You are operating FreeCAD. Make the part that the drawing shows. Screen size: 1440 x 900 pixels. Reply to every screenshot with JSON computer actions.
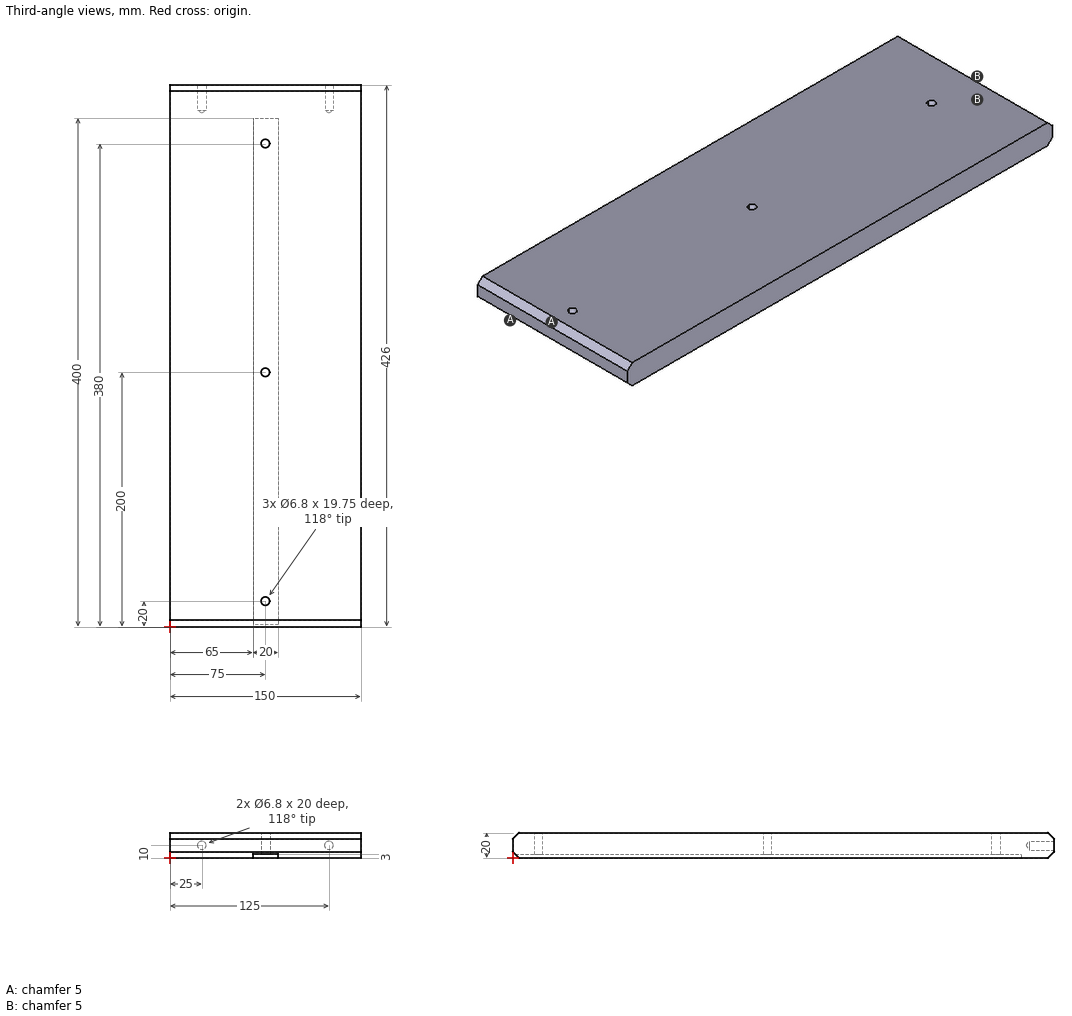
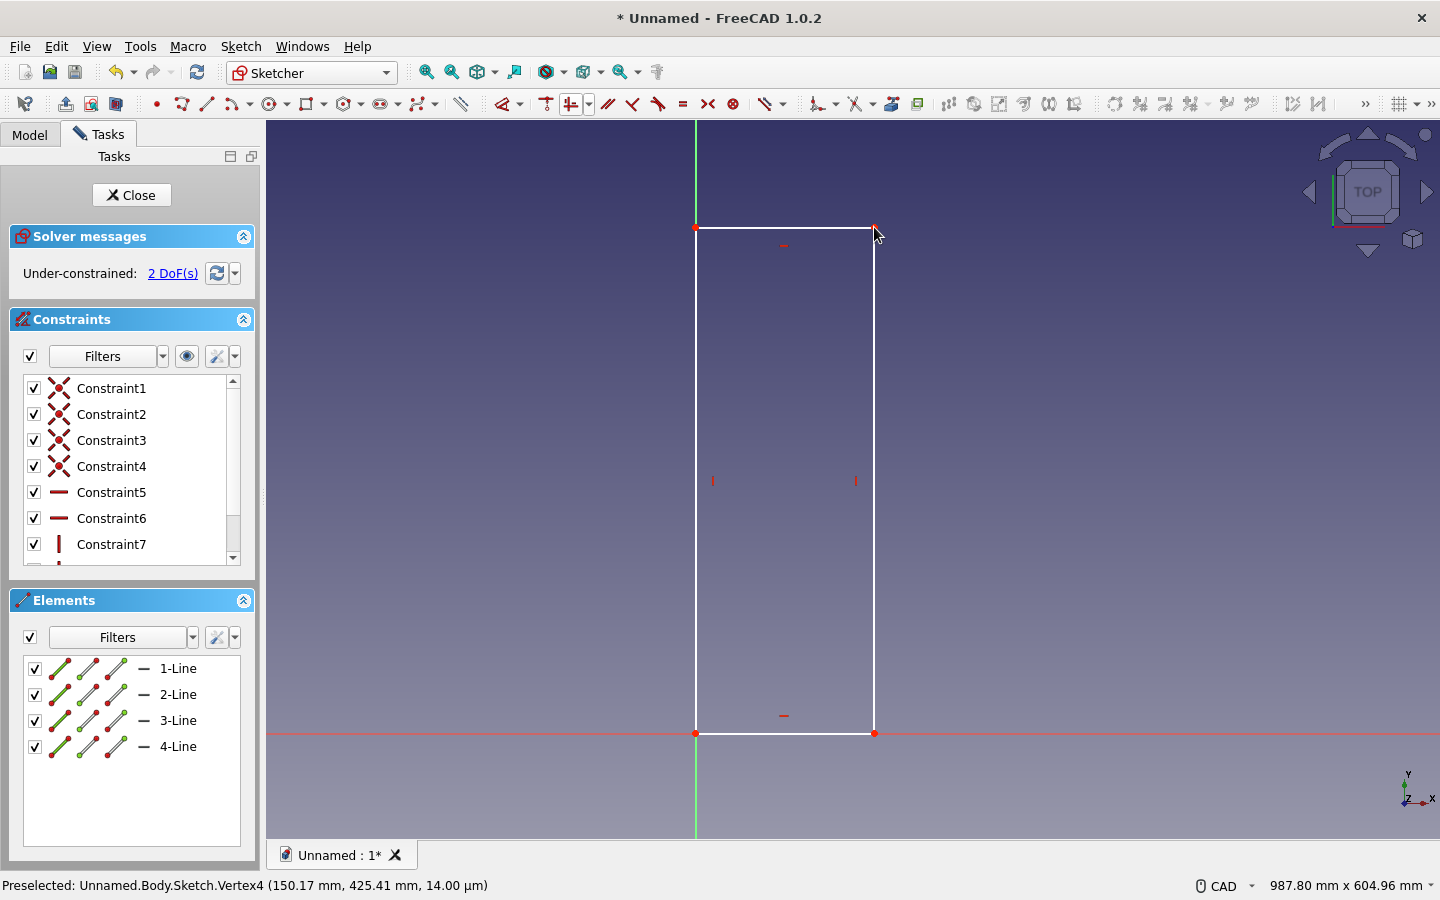
{"action": "key", "text": "d"}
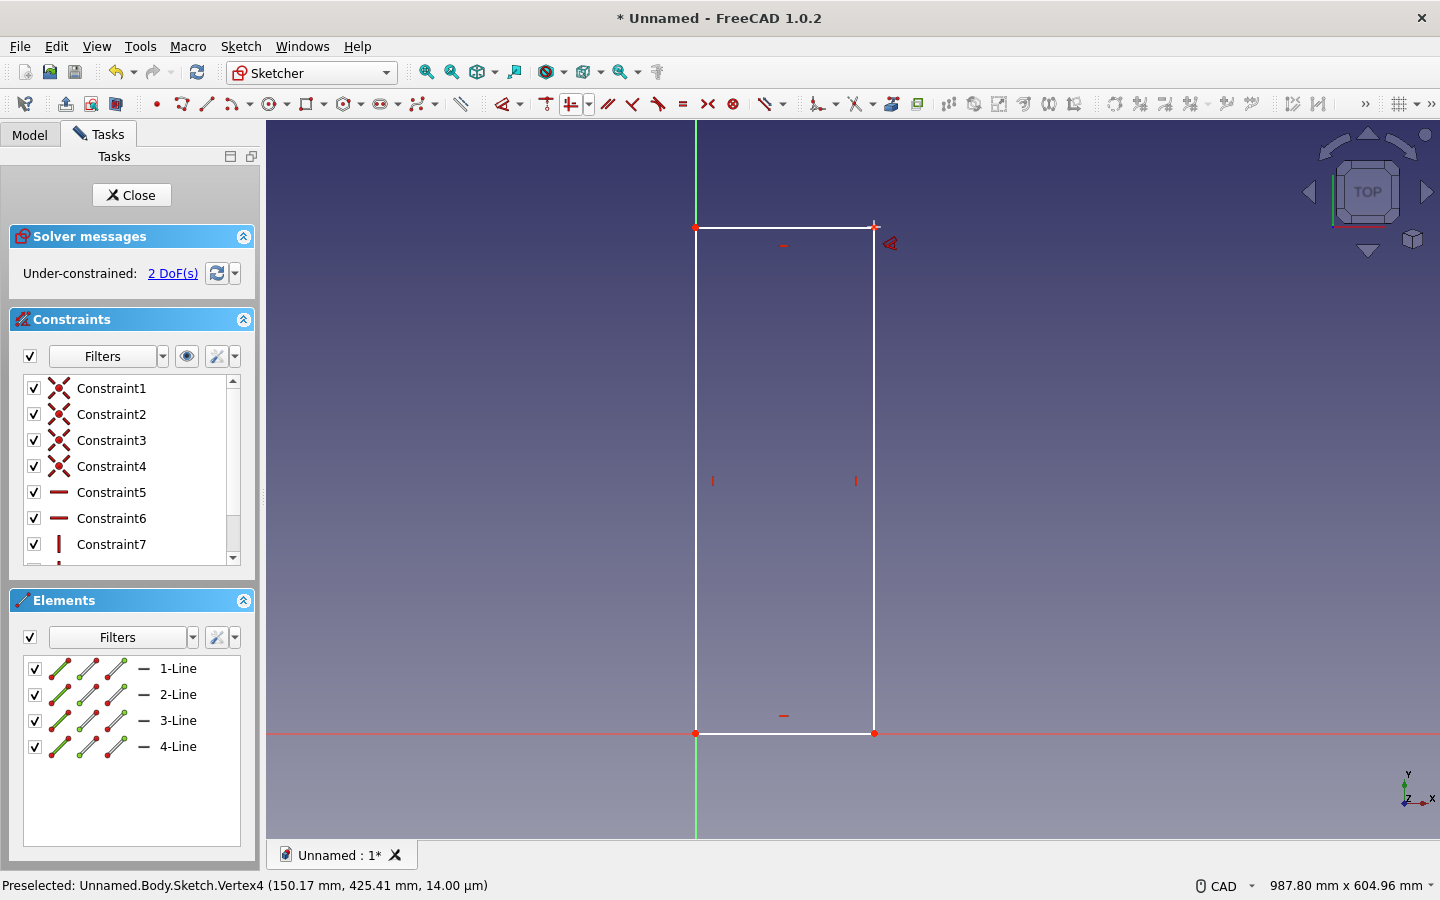
{"action": "left_click", "coordinate": [749, 734]}
{"action": "left_click", "coordinate": [785, 768]}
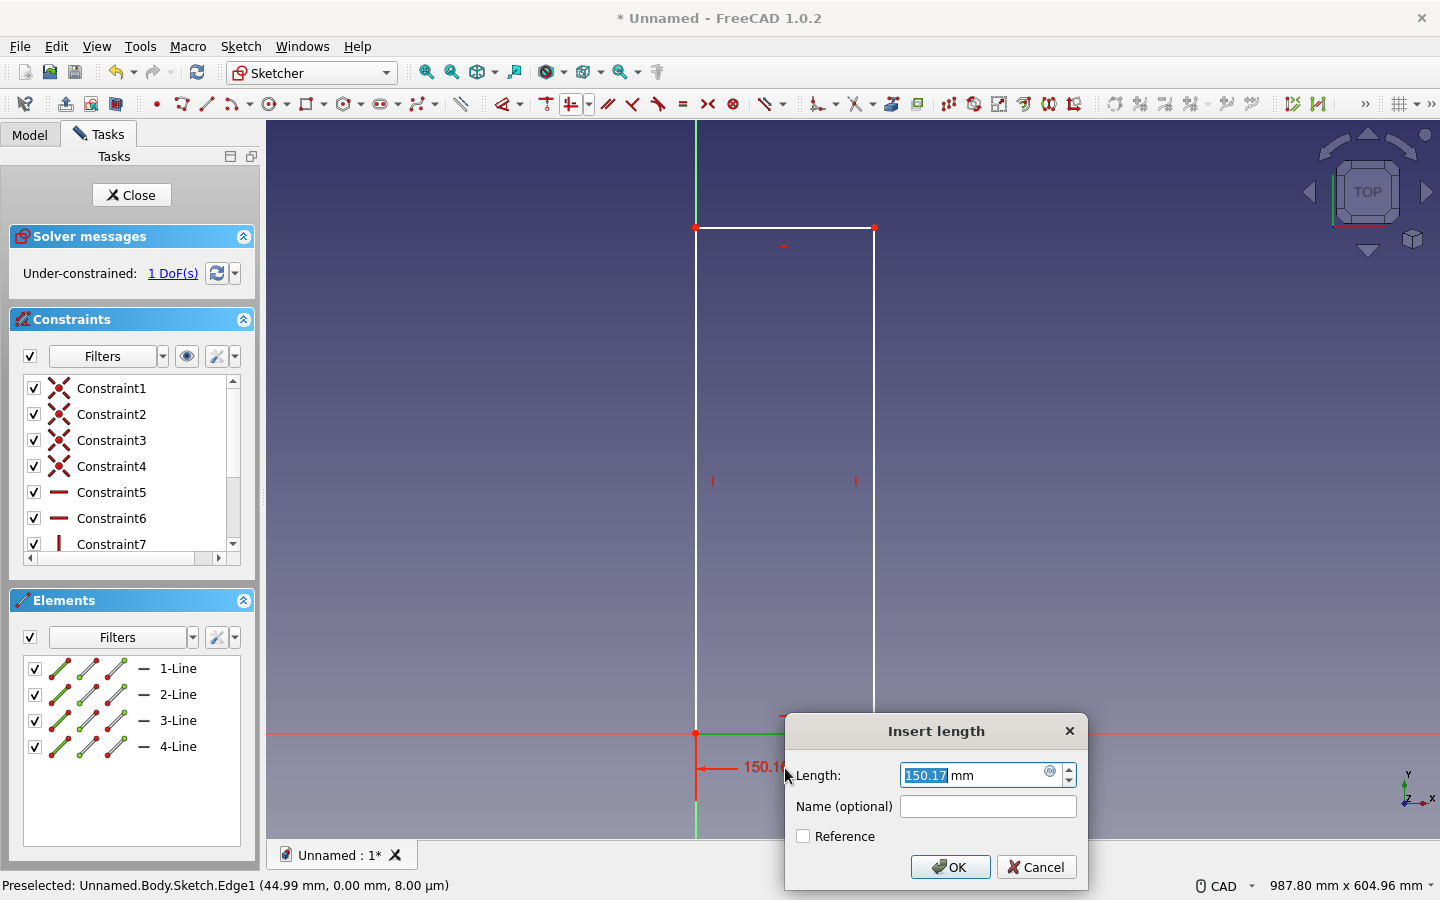
{"action": "type", "text": "150"}
{"action": "key", "text": "Return"}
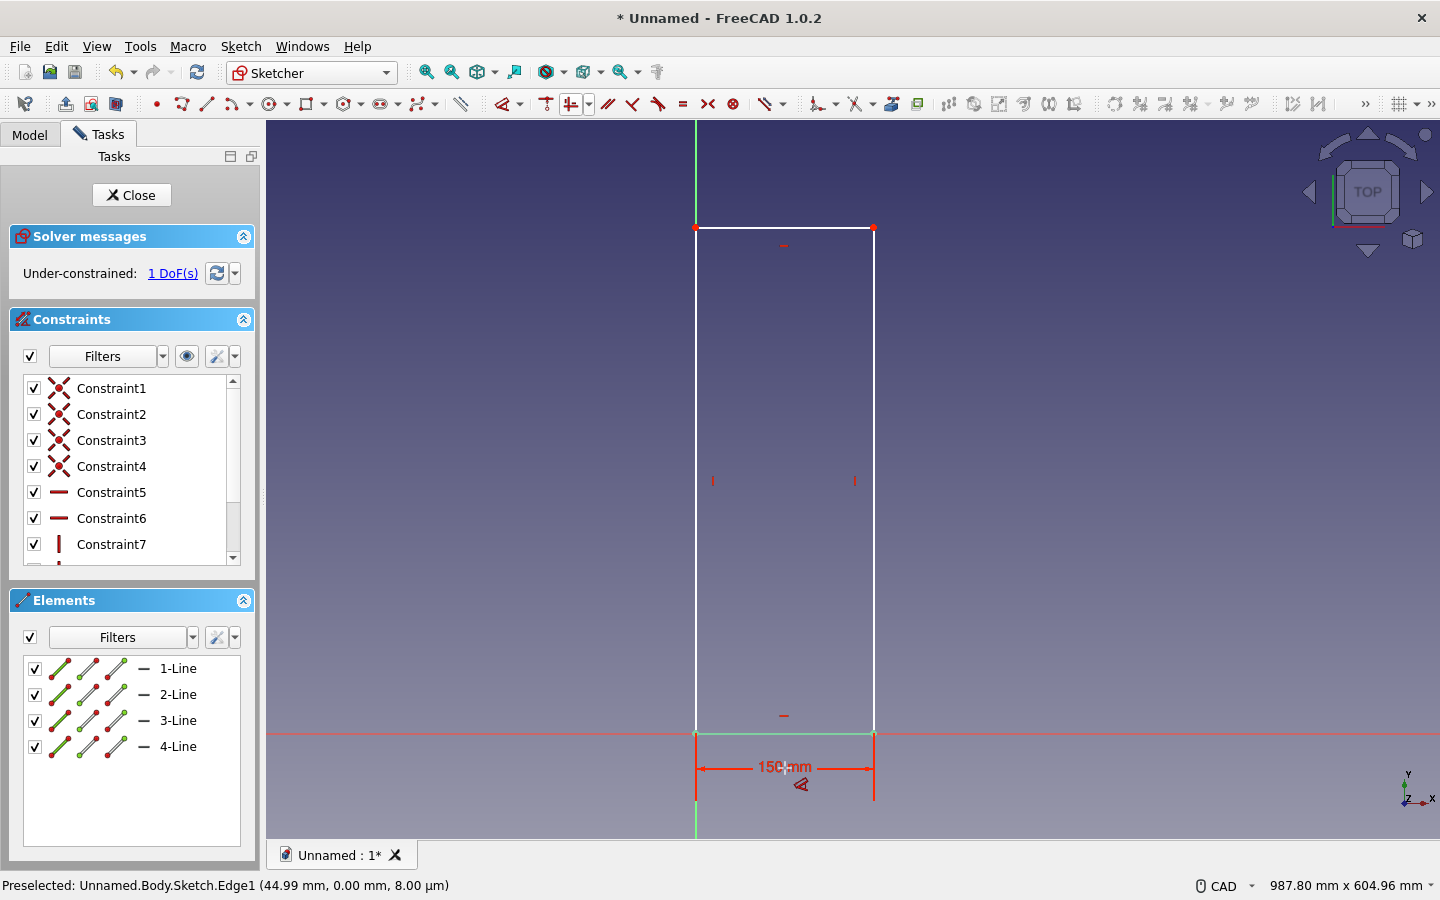
{"action": "left_click", "coordinate": [874, 582]}
{"action": "left_click", "coordinate": [908, 481]}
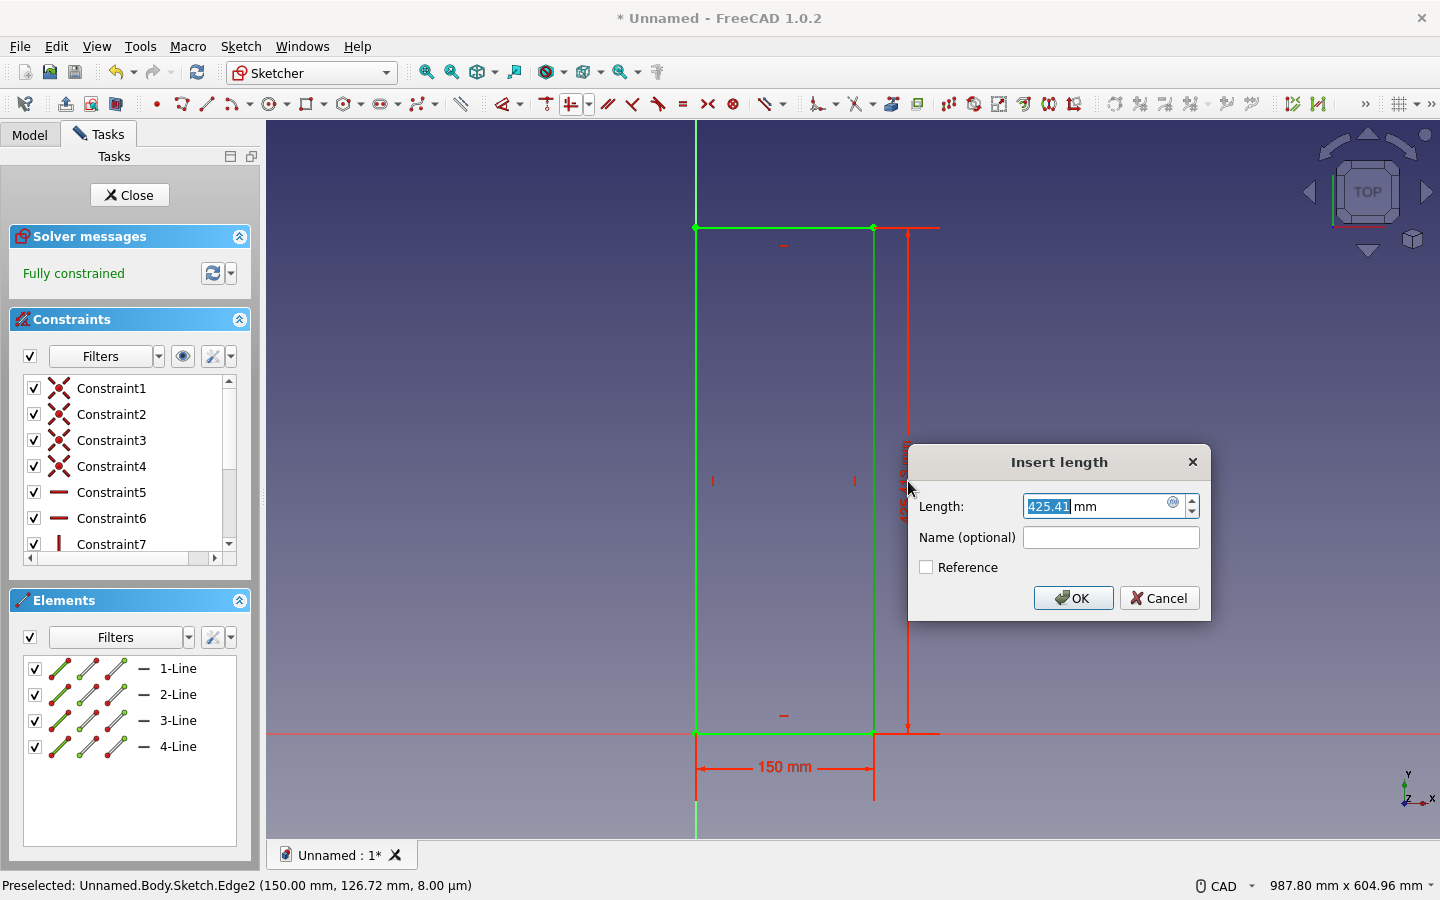
{"action": "type", "text": "426"}
{"action": "key", "text": "Return"}
{"action": "key", "text": "Escape"}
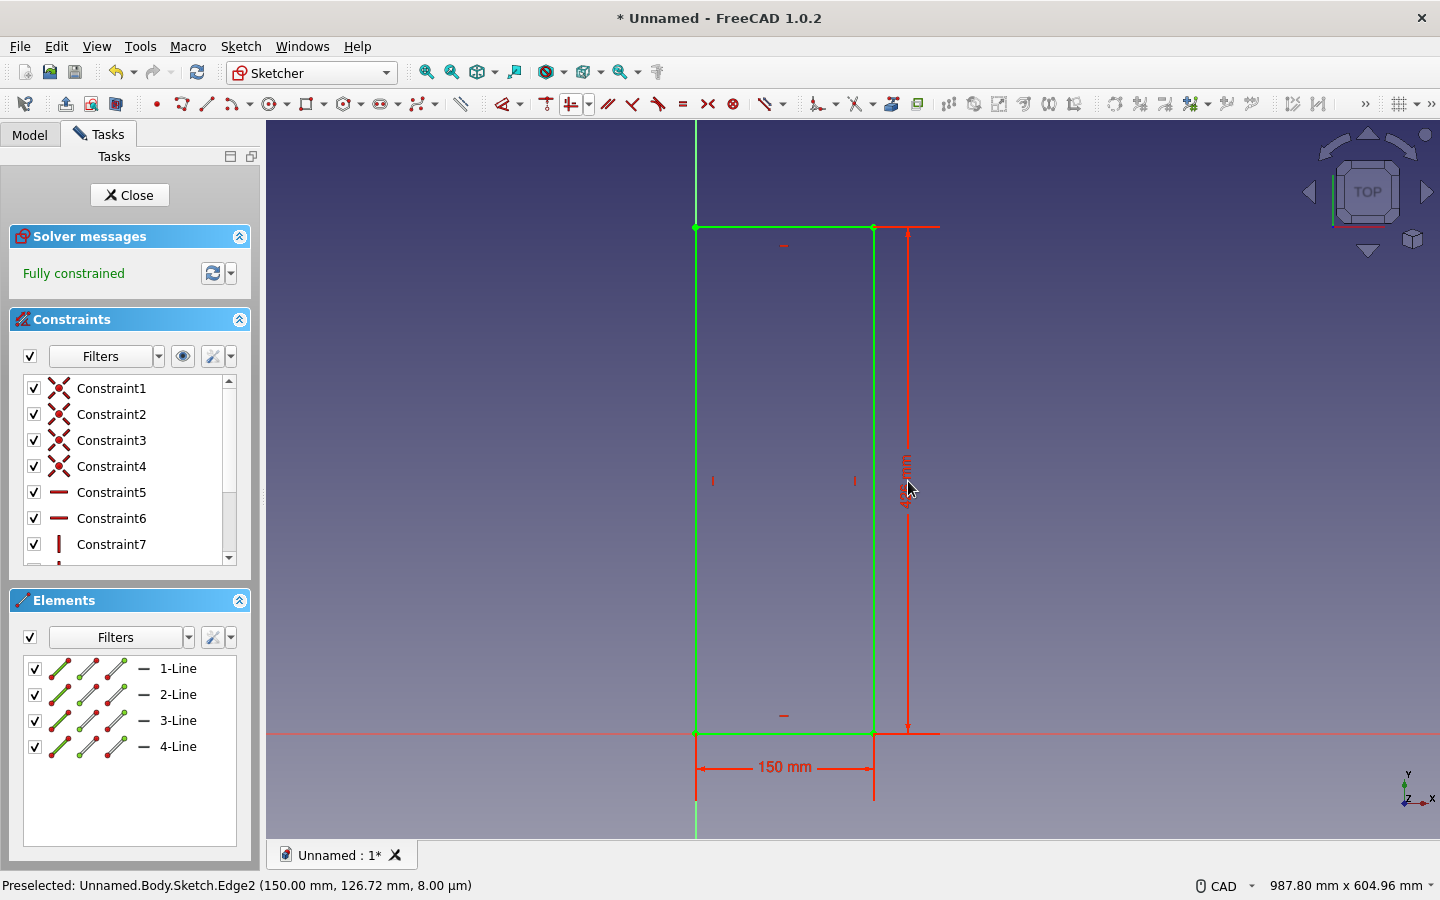
{"action": "left_click", "coordinate": [130, 195]}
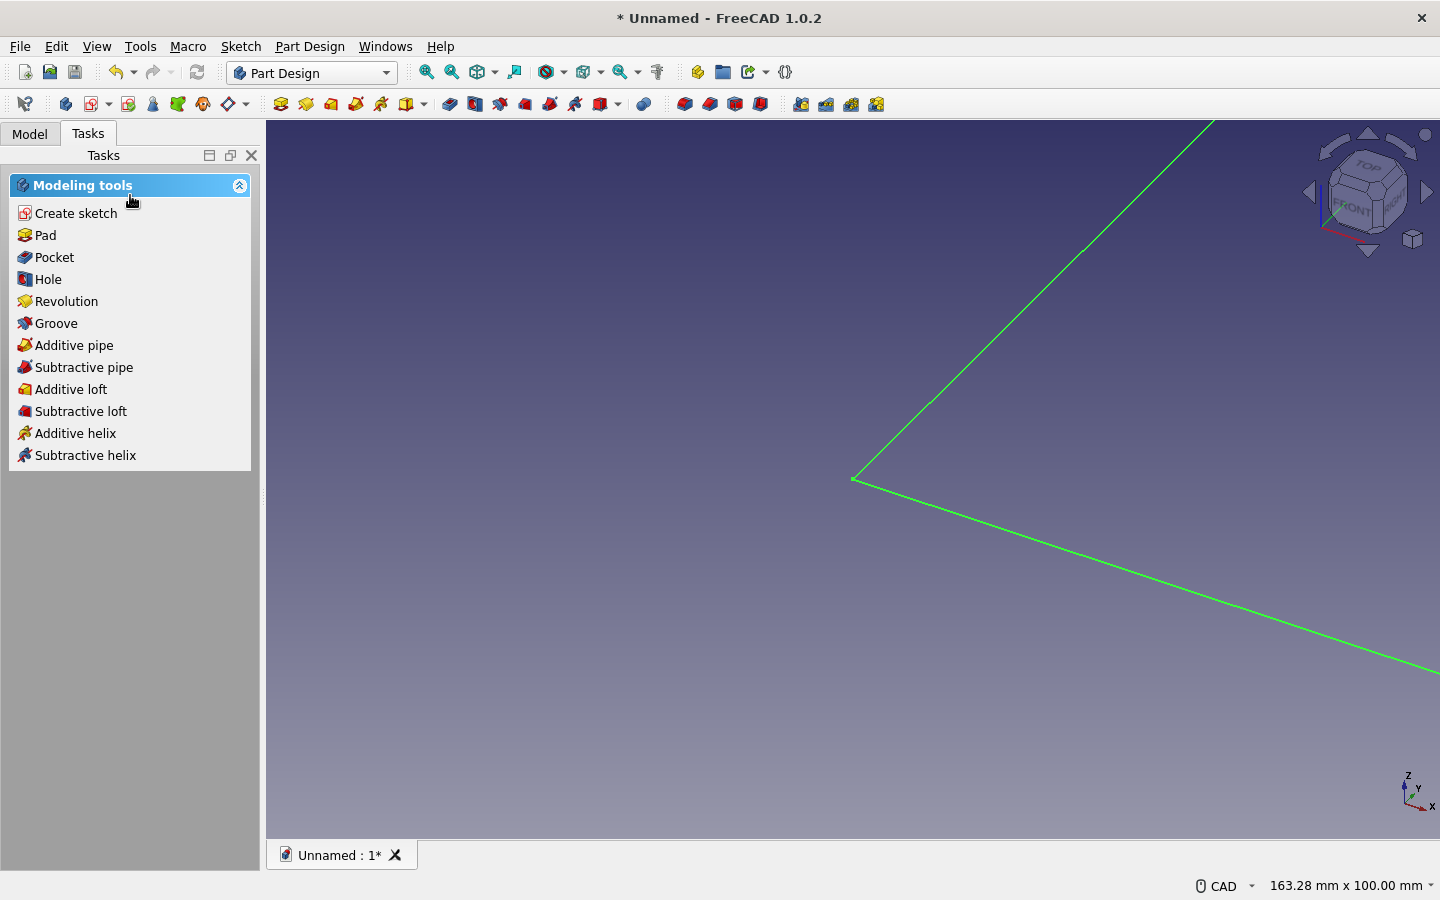
{"action": "left_click", "coordinate": [281, 104]}